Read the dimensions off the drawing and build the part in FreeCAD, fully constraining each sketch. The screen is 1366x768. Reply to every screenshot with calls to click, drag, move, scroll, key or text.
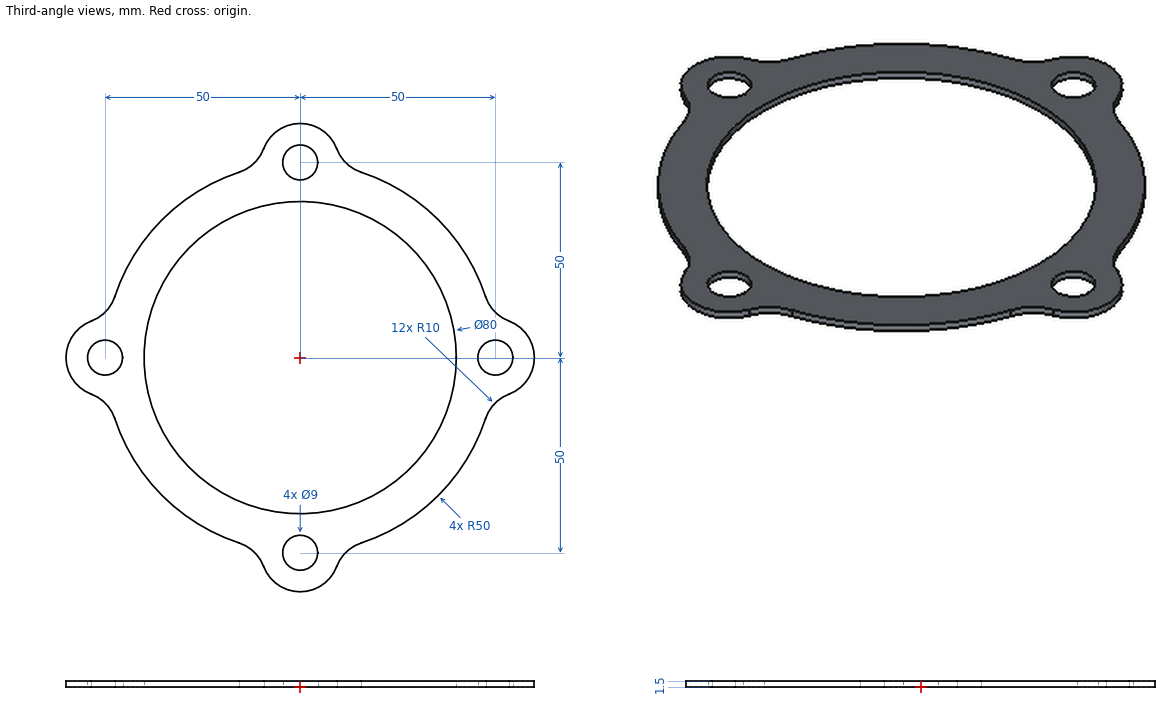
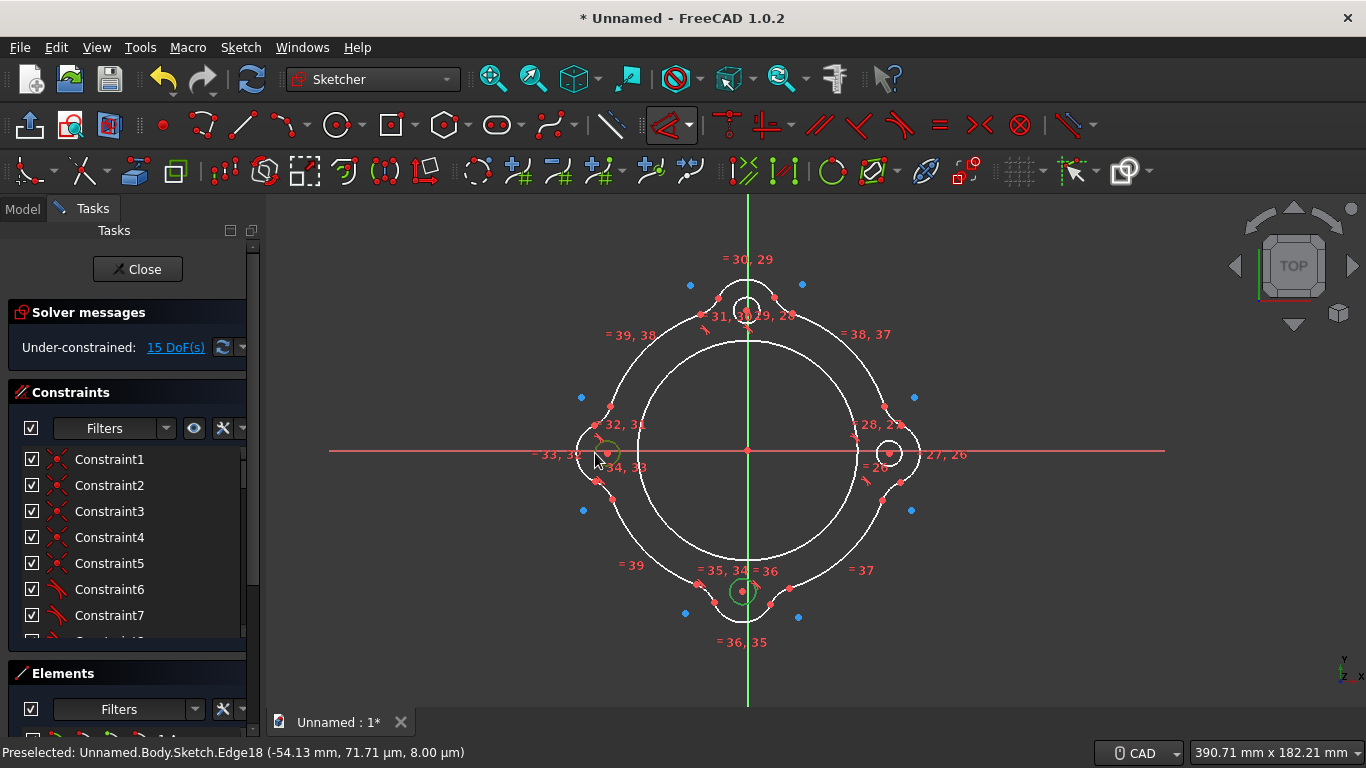
click(898, 462)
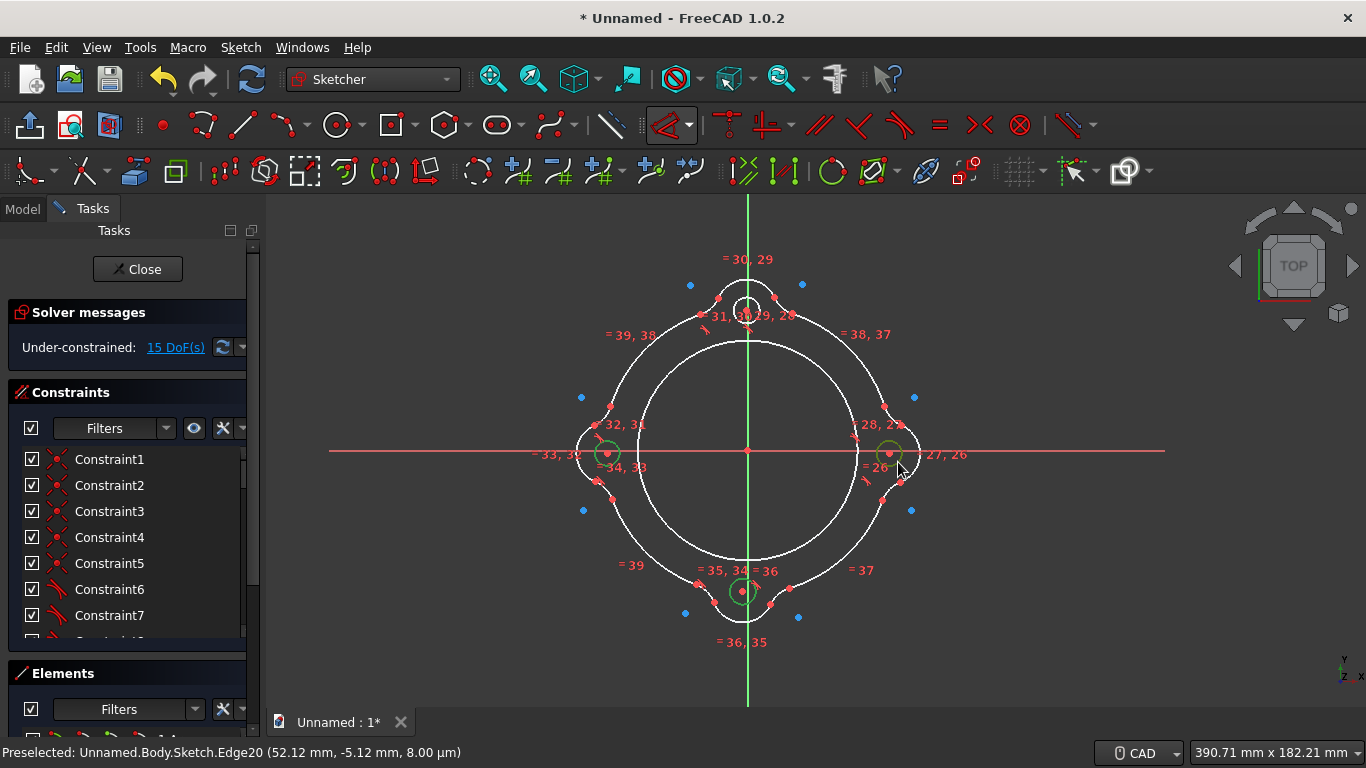
scroll(737, 301, up, 2)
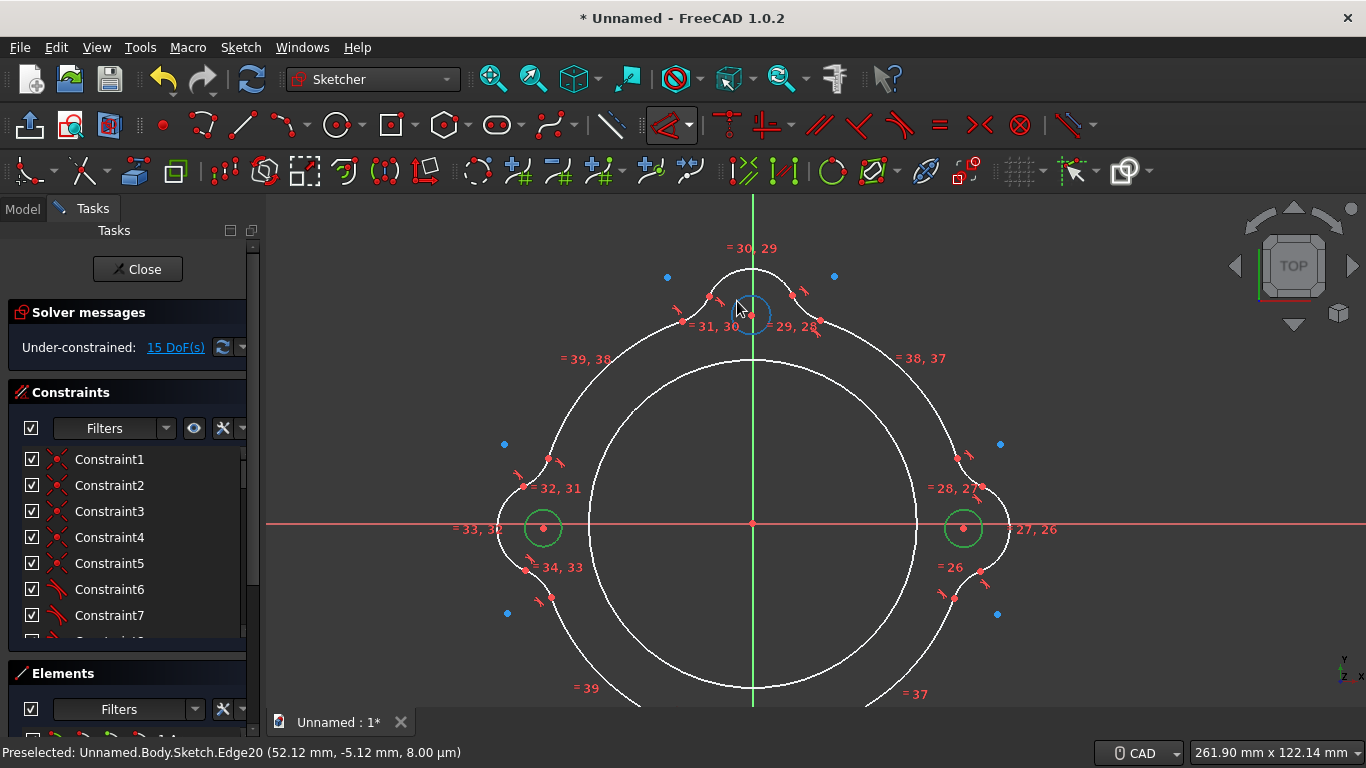
click(737, 301)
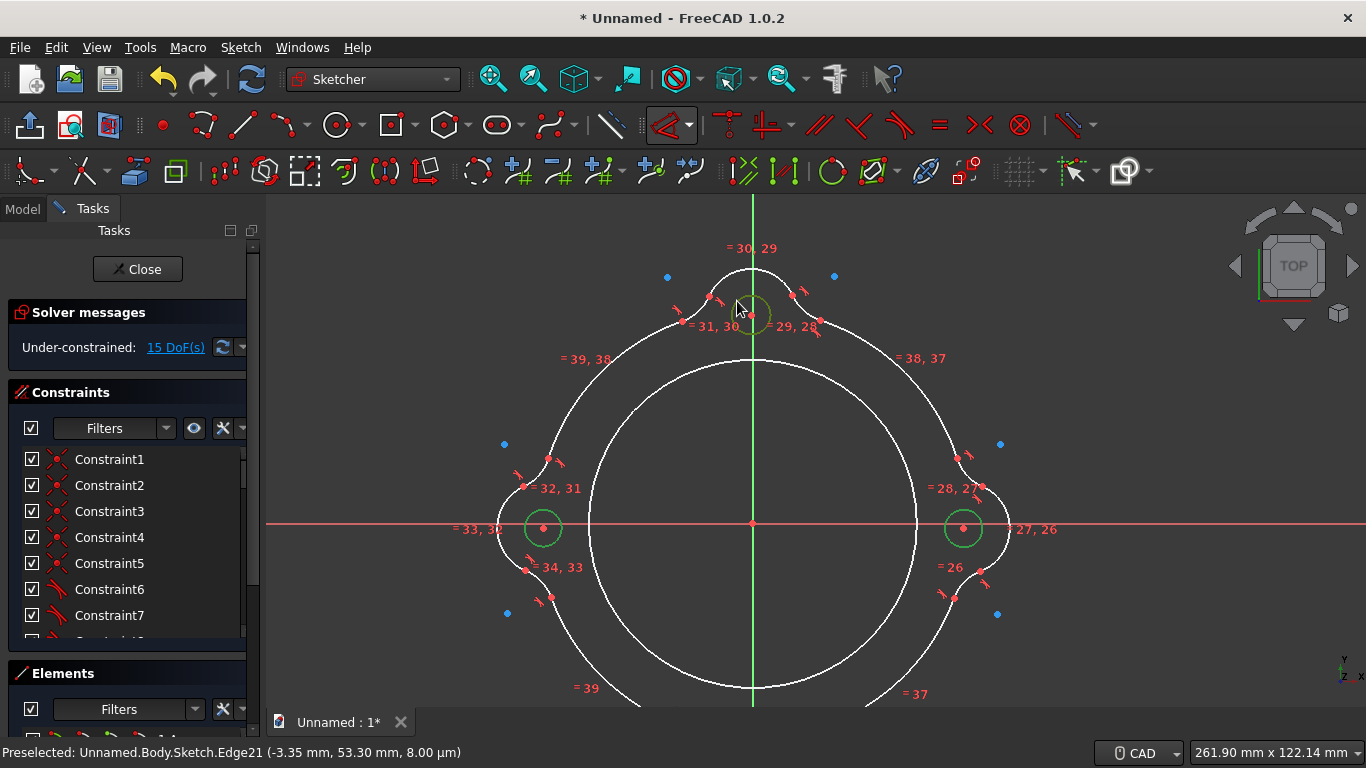
click(940, 126)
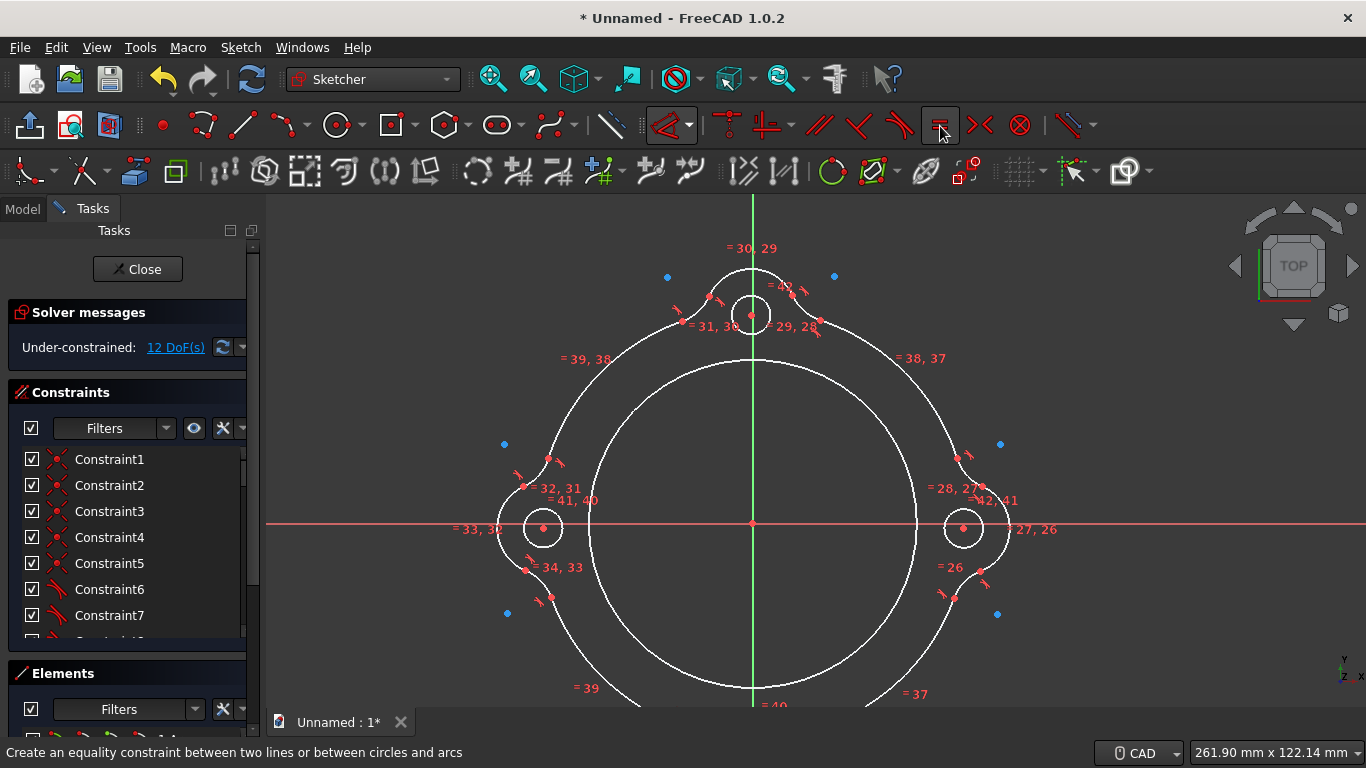
click(964, 528)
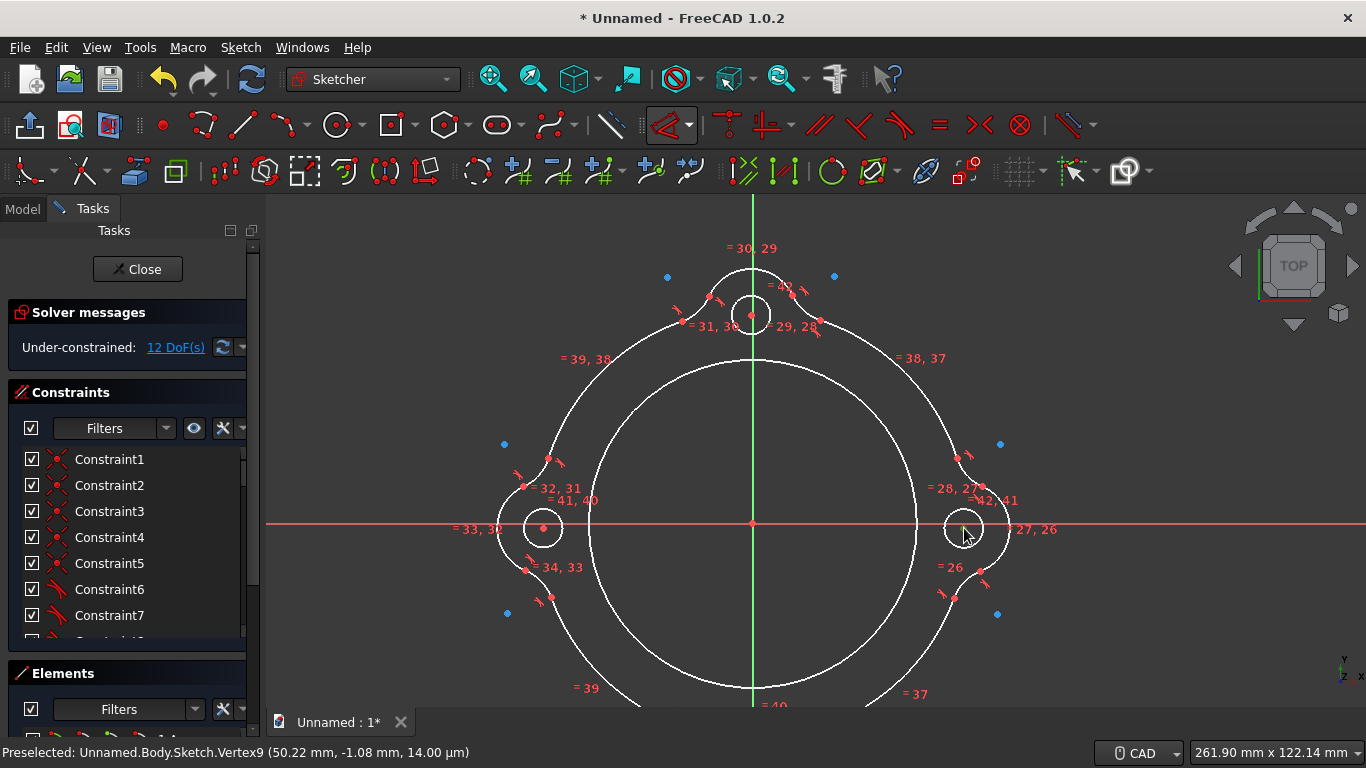
click(359, 524)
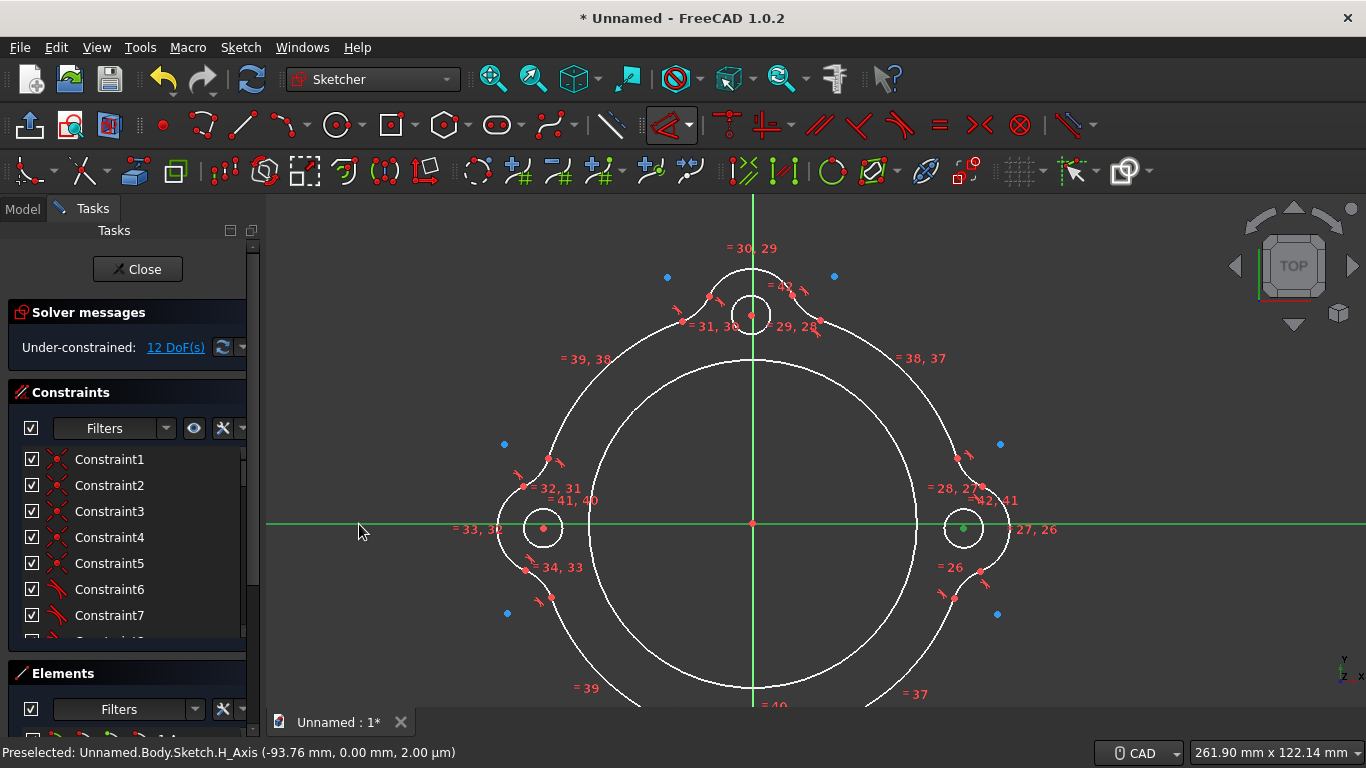
click(728, 126)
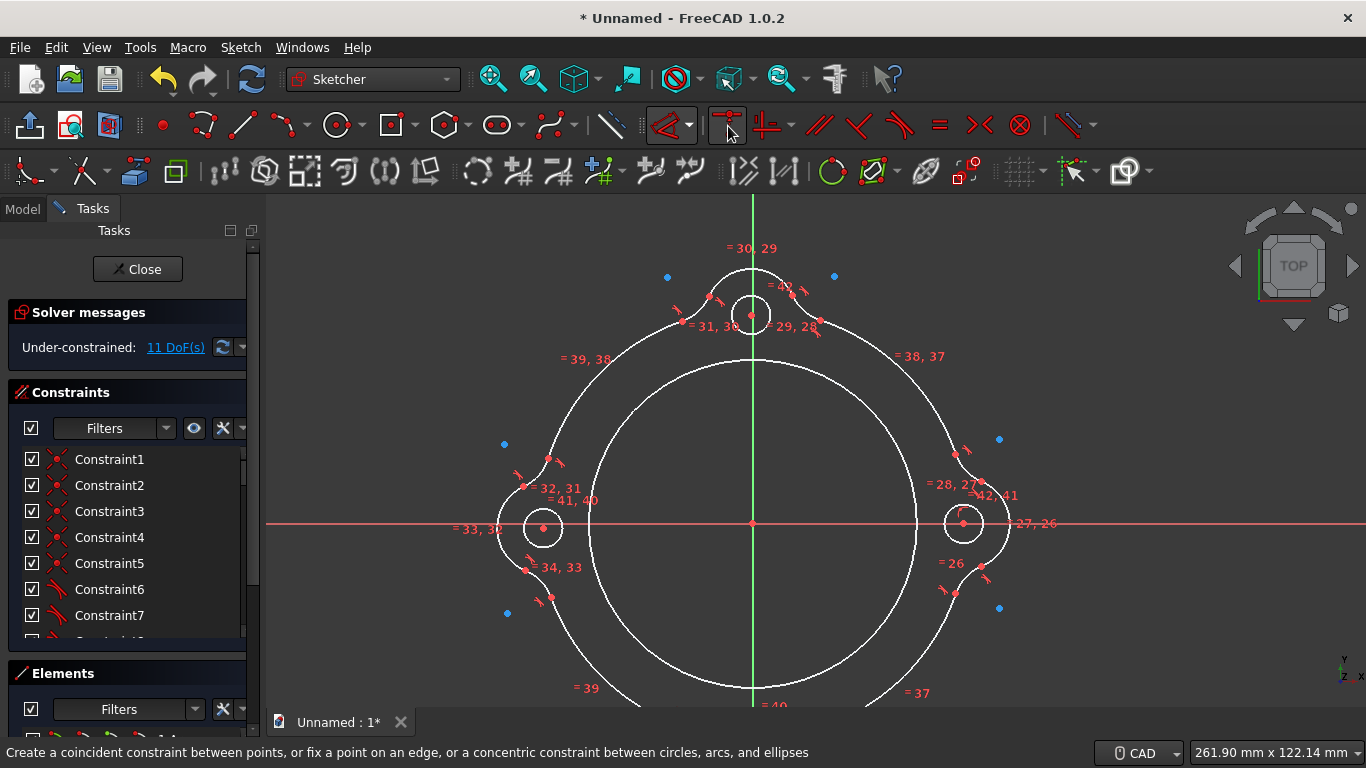
click(751, 315)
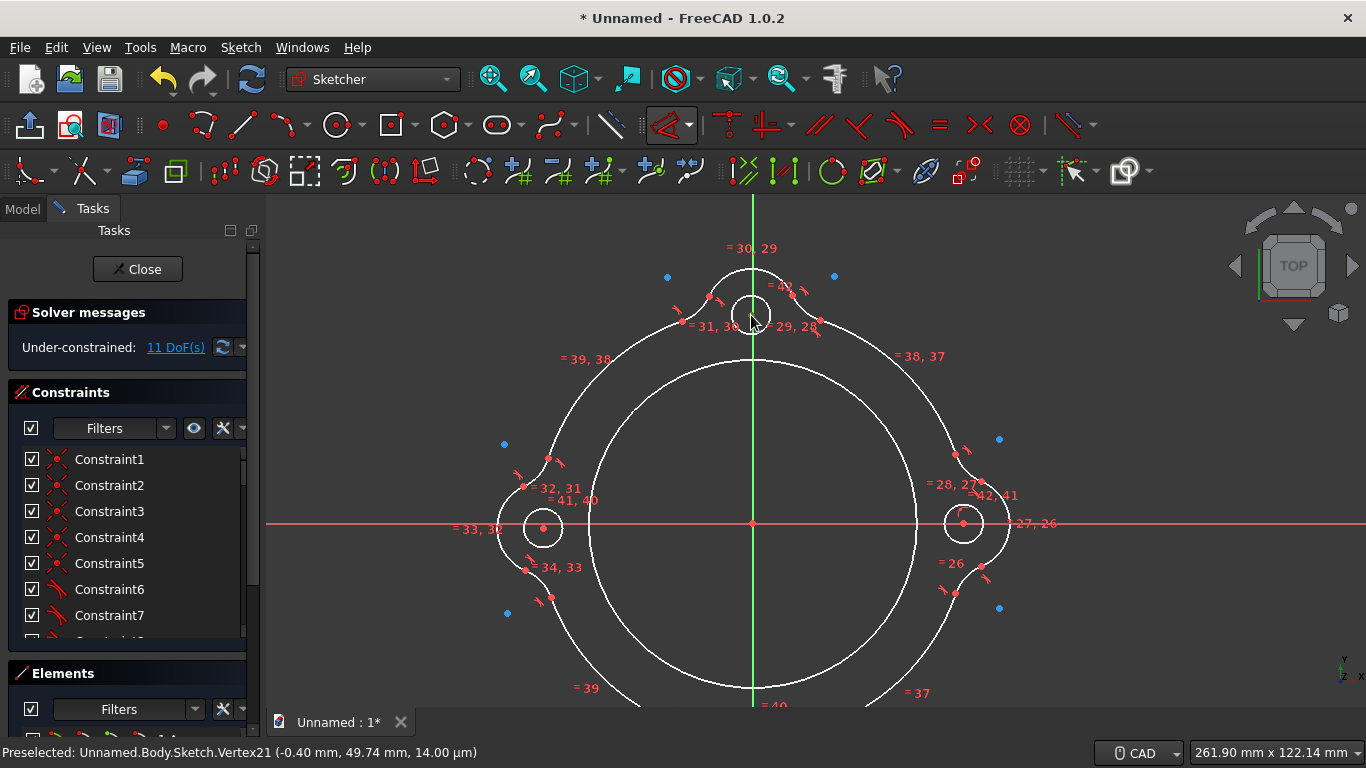
click(753, 646)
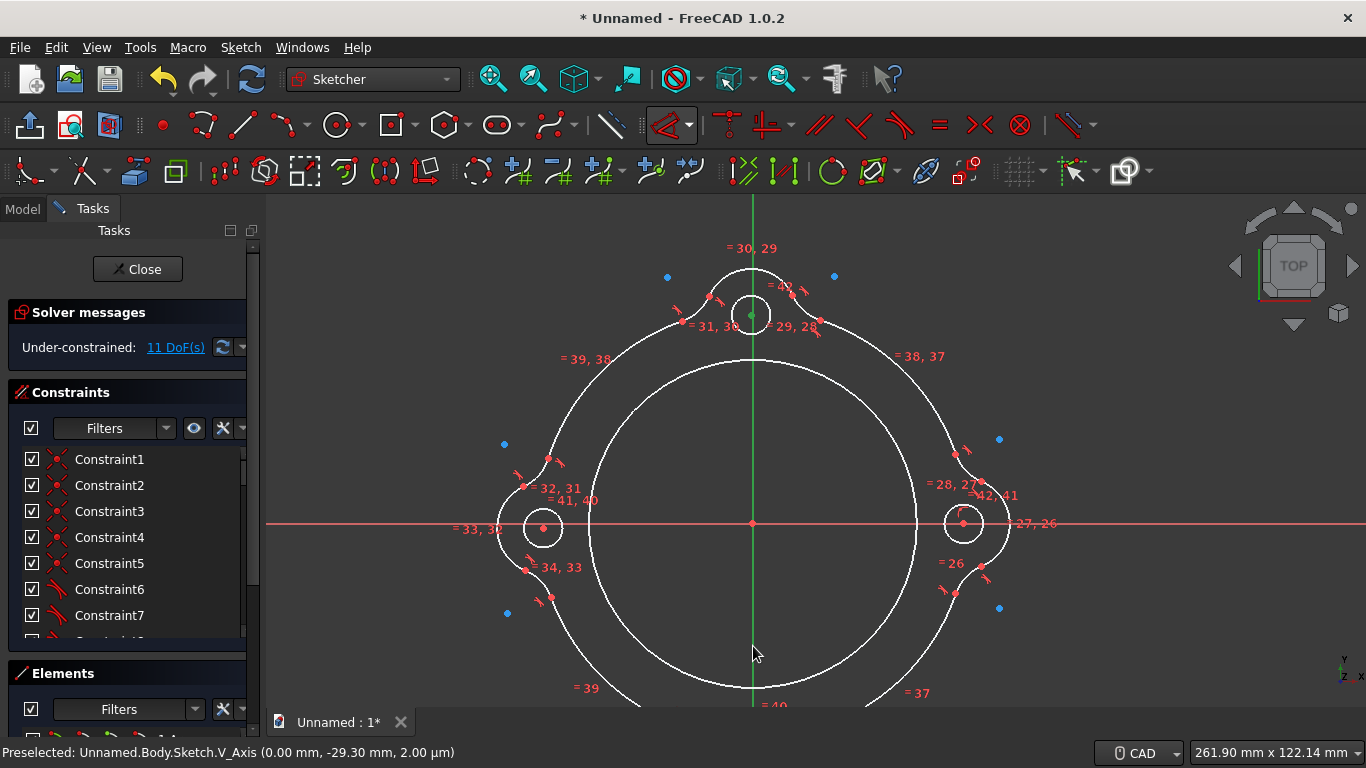
click(728, 126)